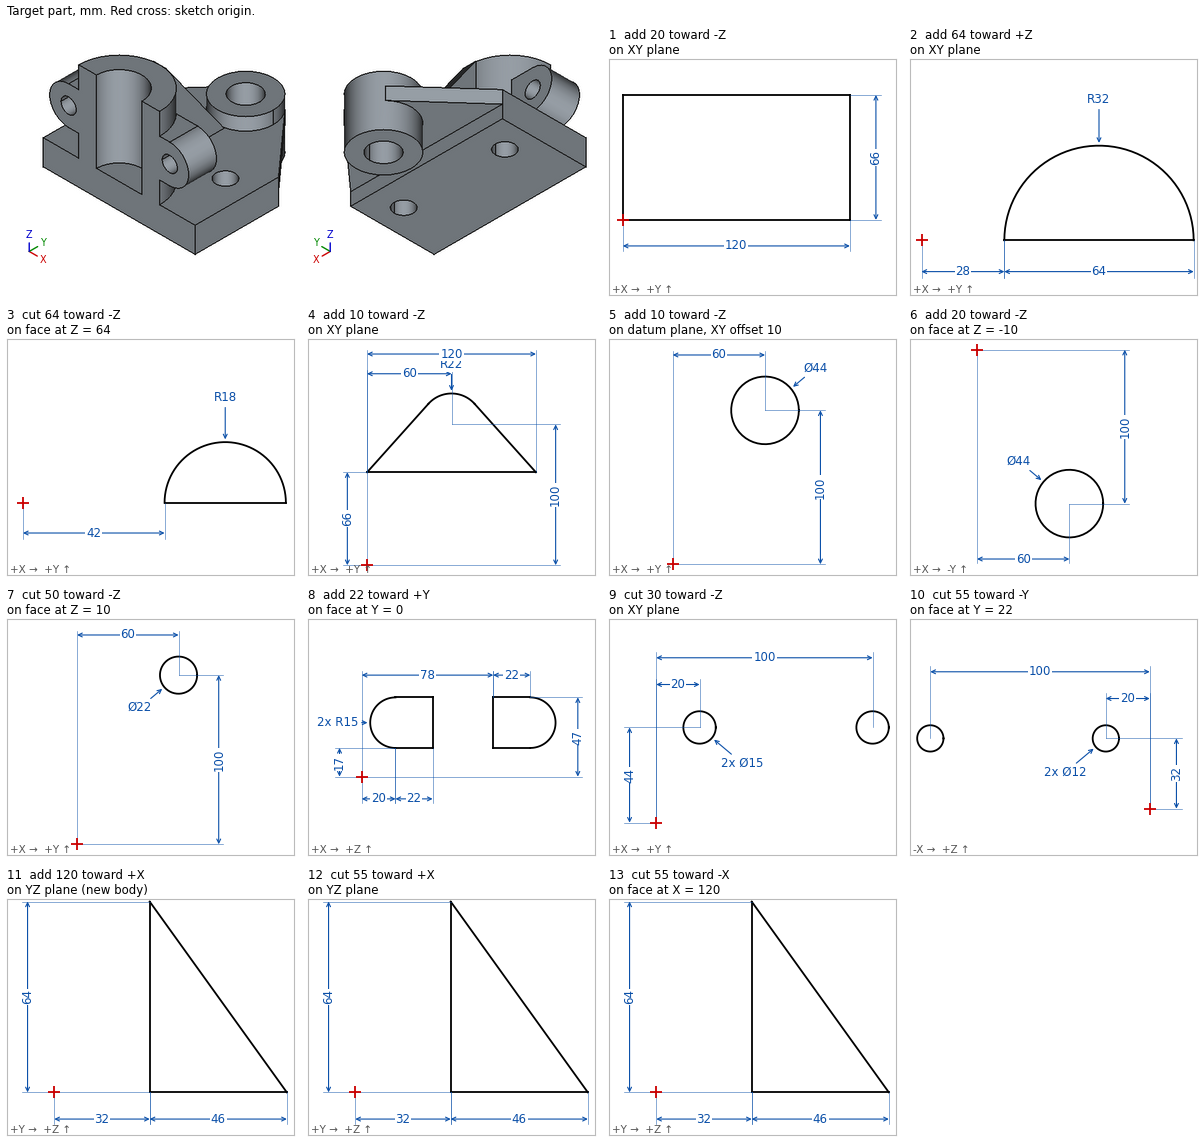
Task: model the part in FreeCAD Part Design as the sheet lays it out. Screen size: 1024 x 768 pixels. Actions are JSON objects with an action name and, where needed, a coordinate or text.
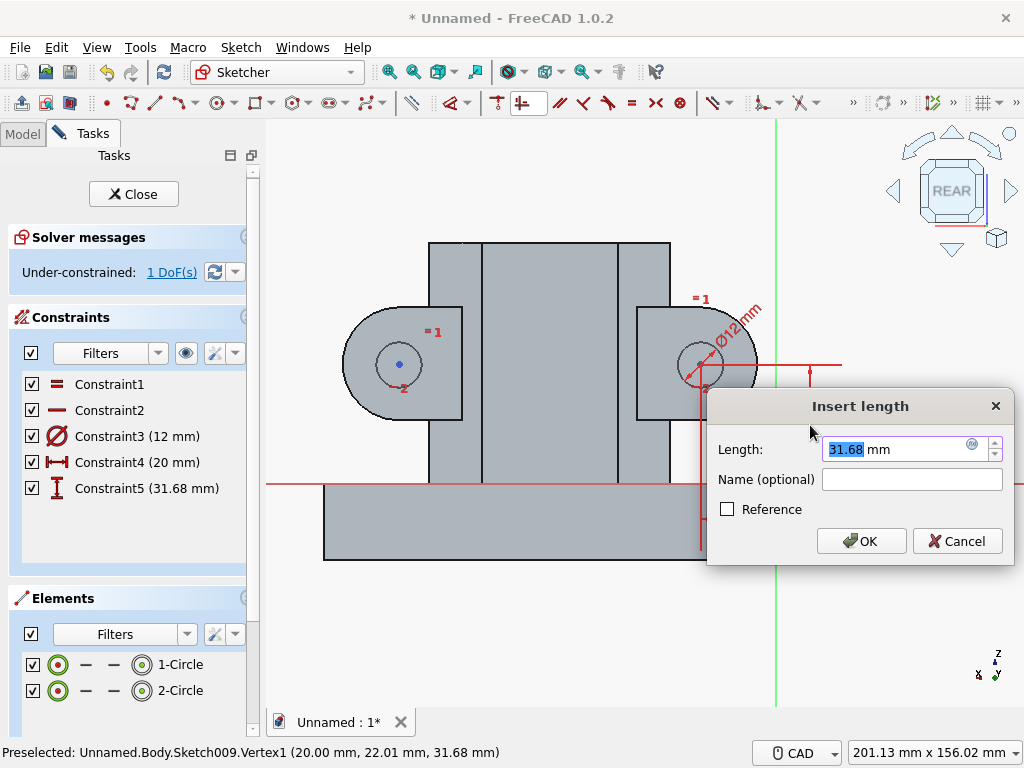
{"action": "type", "text": "32"}
{"action": "key", "text": "Return"}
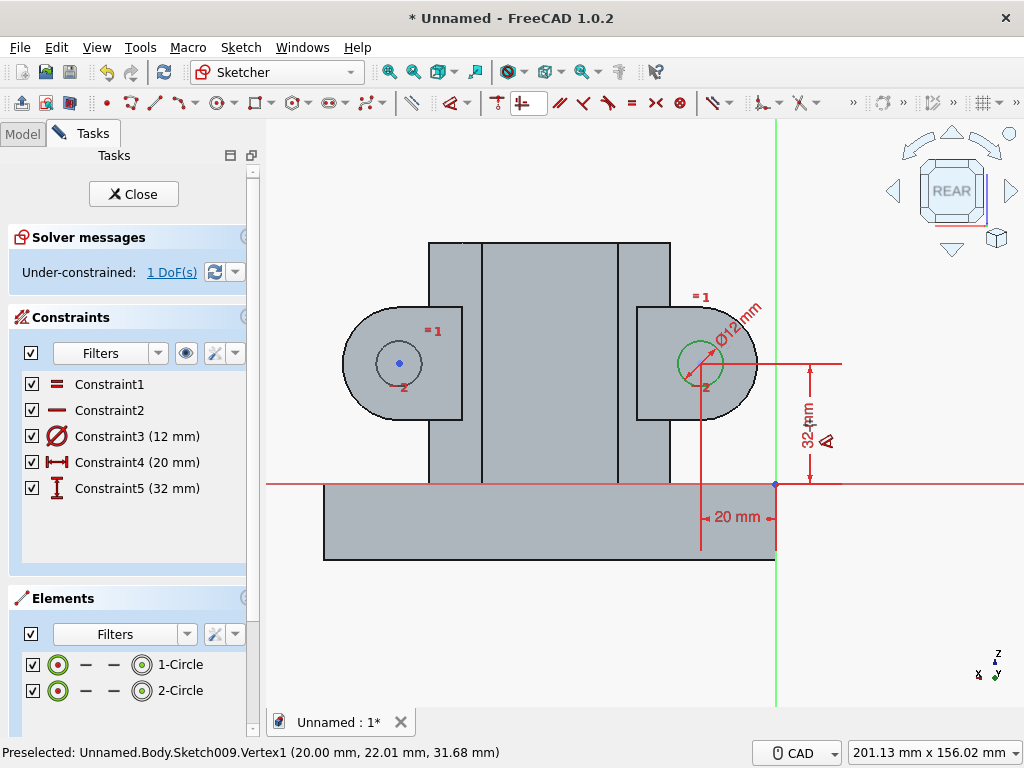
{"action": "left_click", "coordinate": [399, 364]}
{"action": "left_click", "coordinate": [587, 518]}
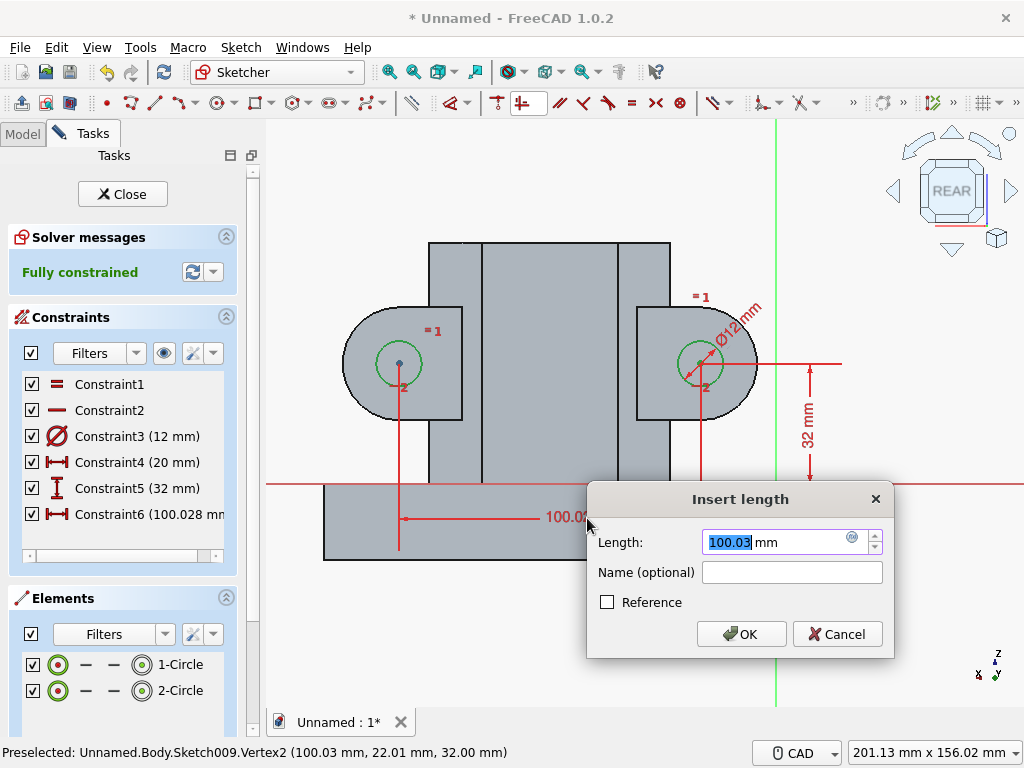
{"action": "type", "text": "100"}
{"action": "key", "text": "Return"}
{"action": "key", "text": "Escape"}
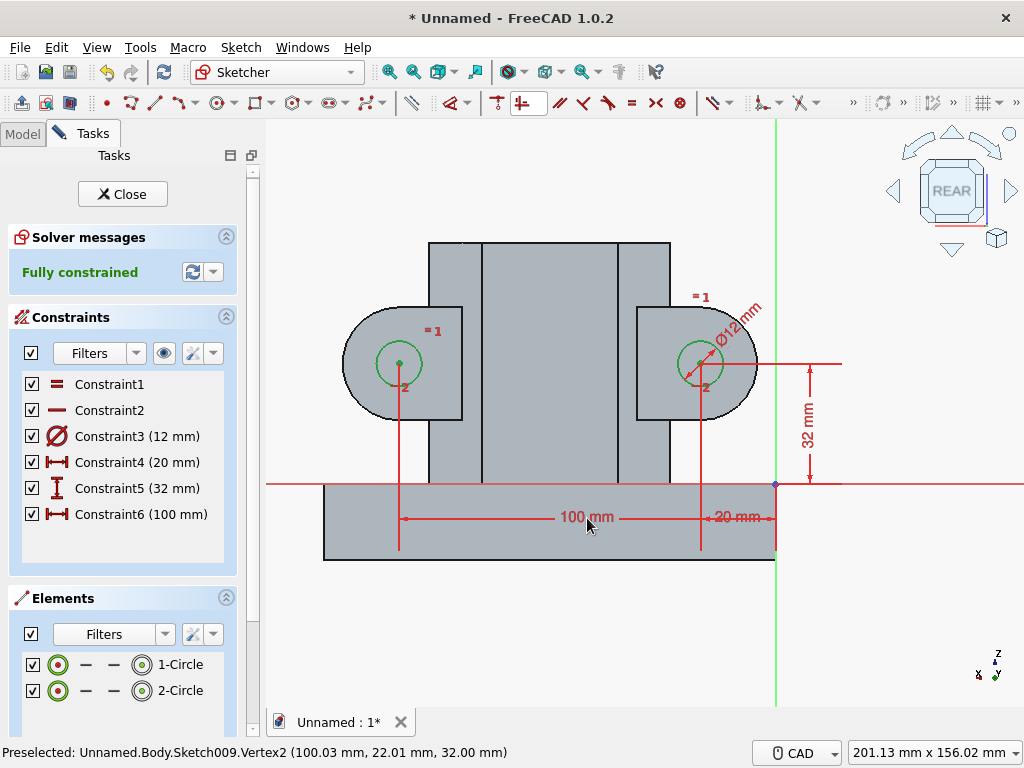
{"action": "left_click", "coordinate": [123, 194]}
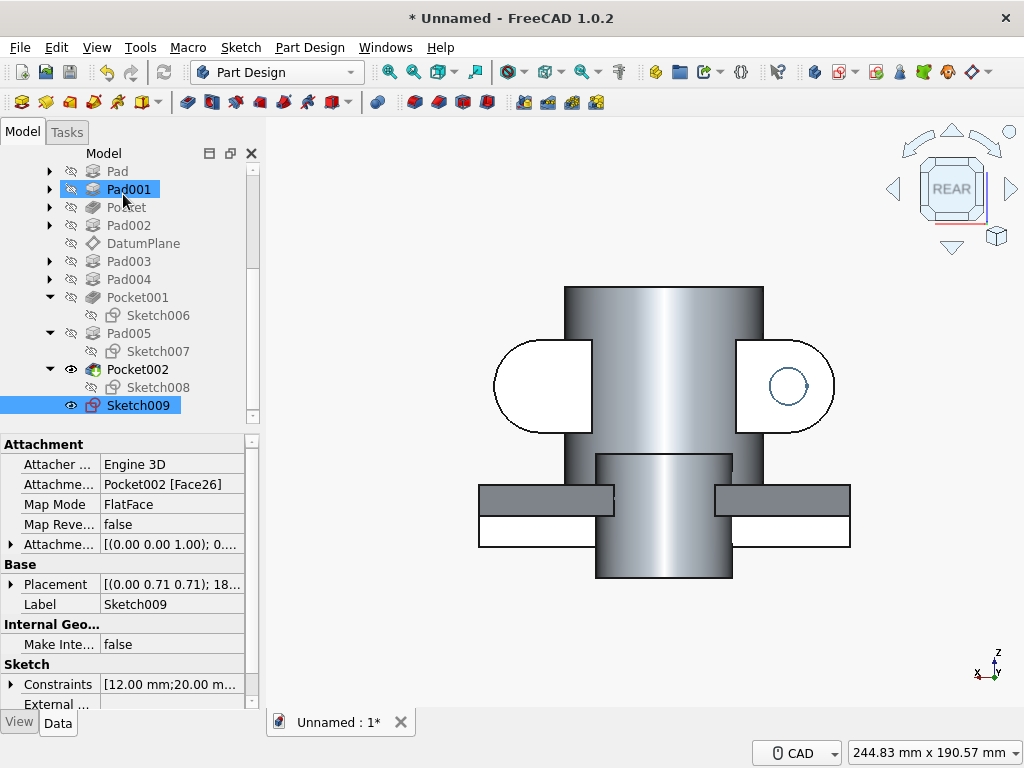
{"action": "left_click", "coordinate": [188, 102]}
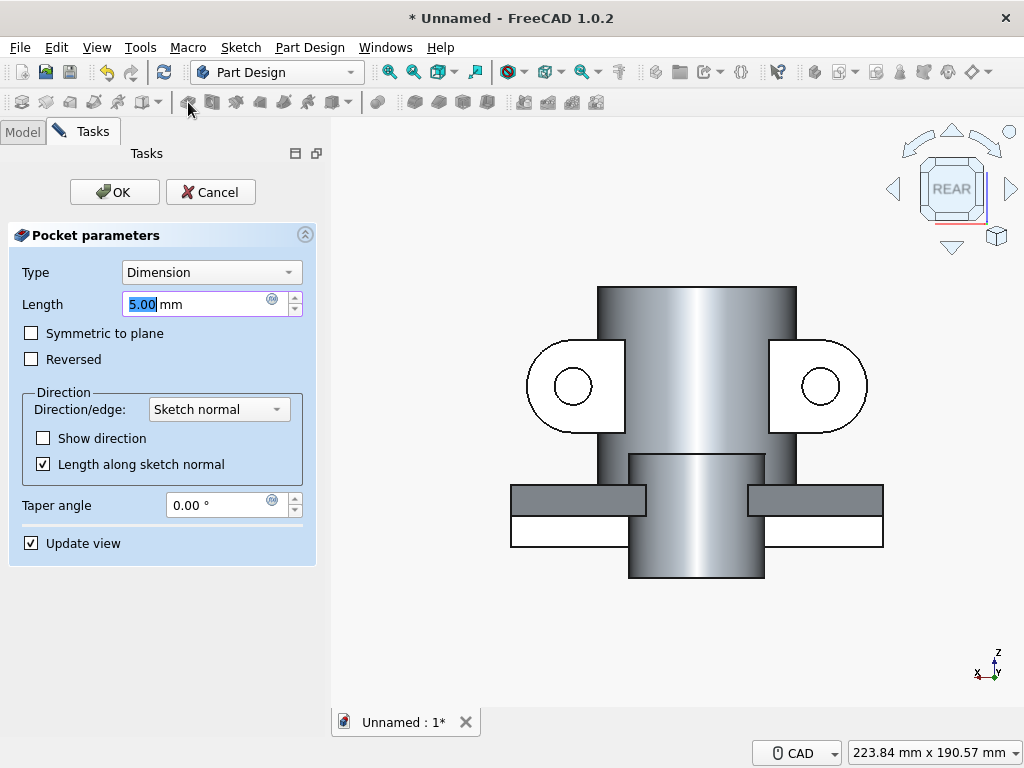
{"action": "type", "text": "55"}
{"action": "key", "text": "Tab"}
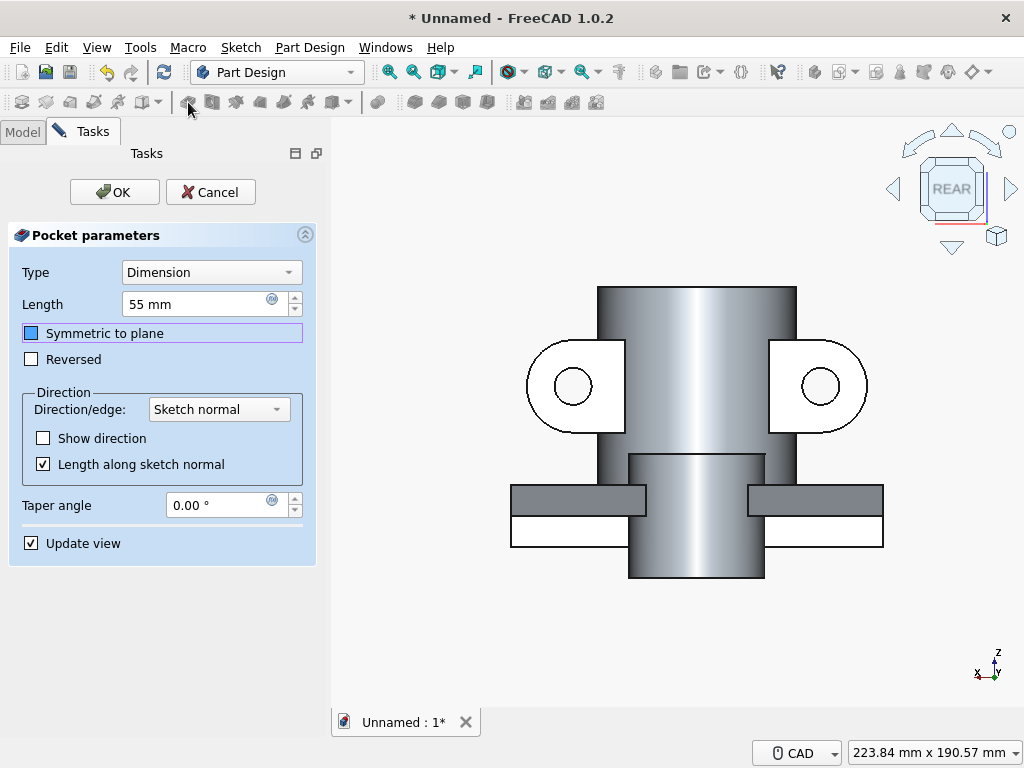
{"action": "left_click", "coordinate": [115, 192]}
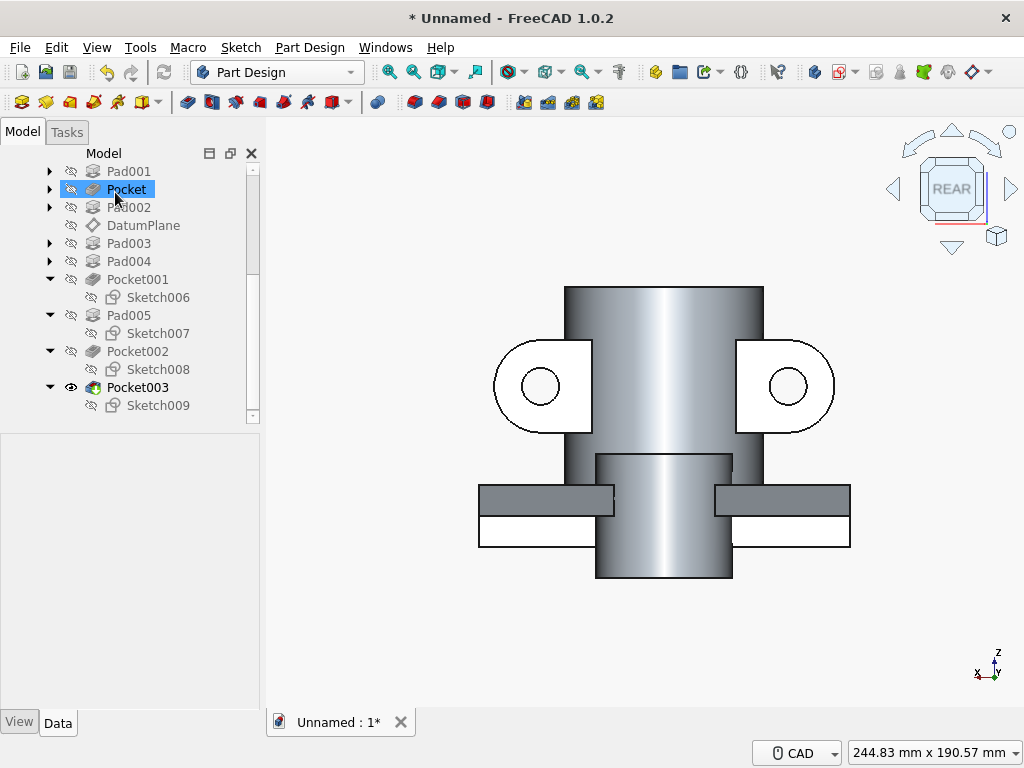
{"action": "left_click", "coordinate": [816, 72]}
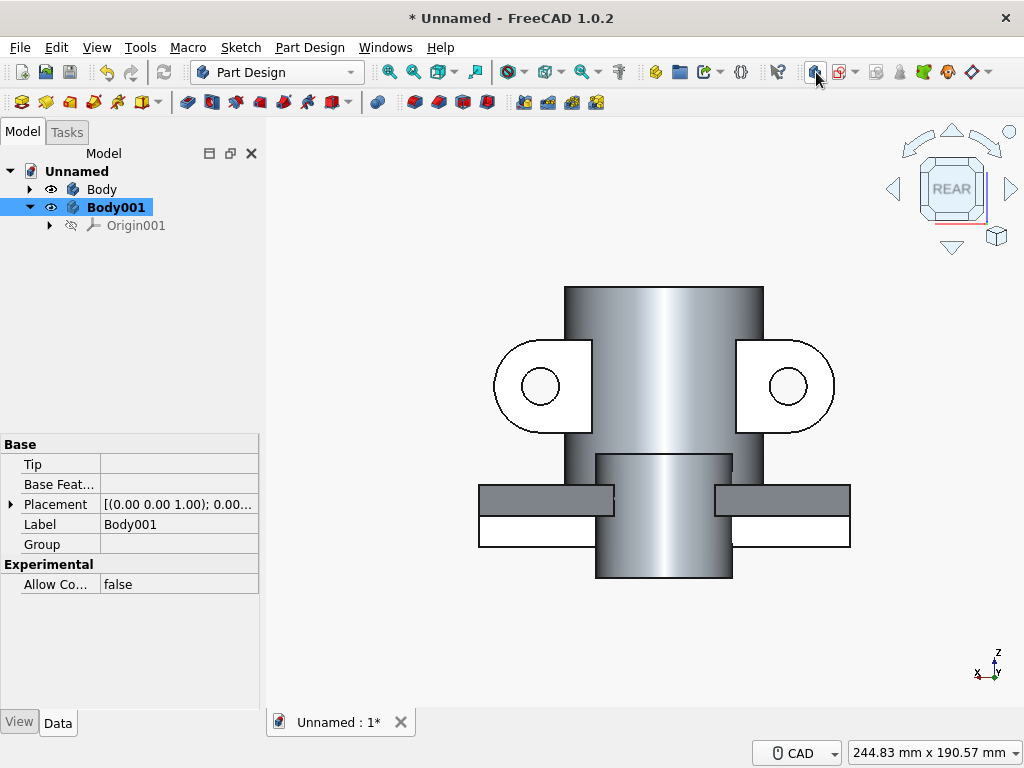
{"action": "left_click", "coordinate": [306, 667]}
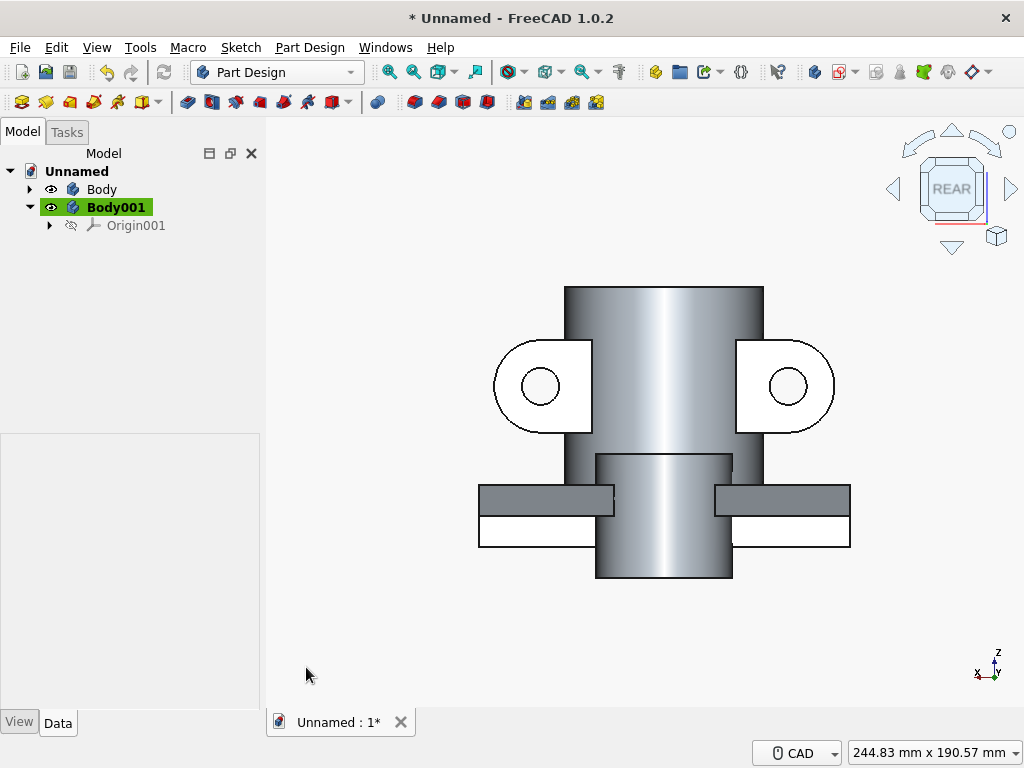
{"action": "left_click", "coordinate": [840, 72]}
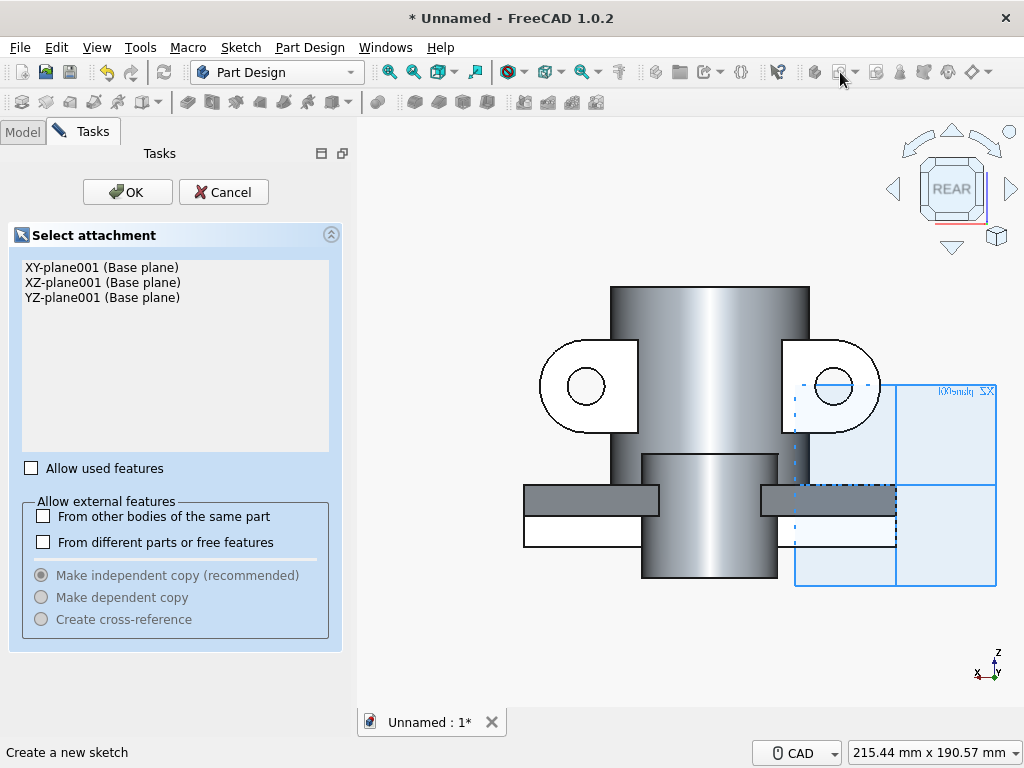
{"action": "left_click", "coordinate": [82, 298]}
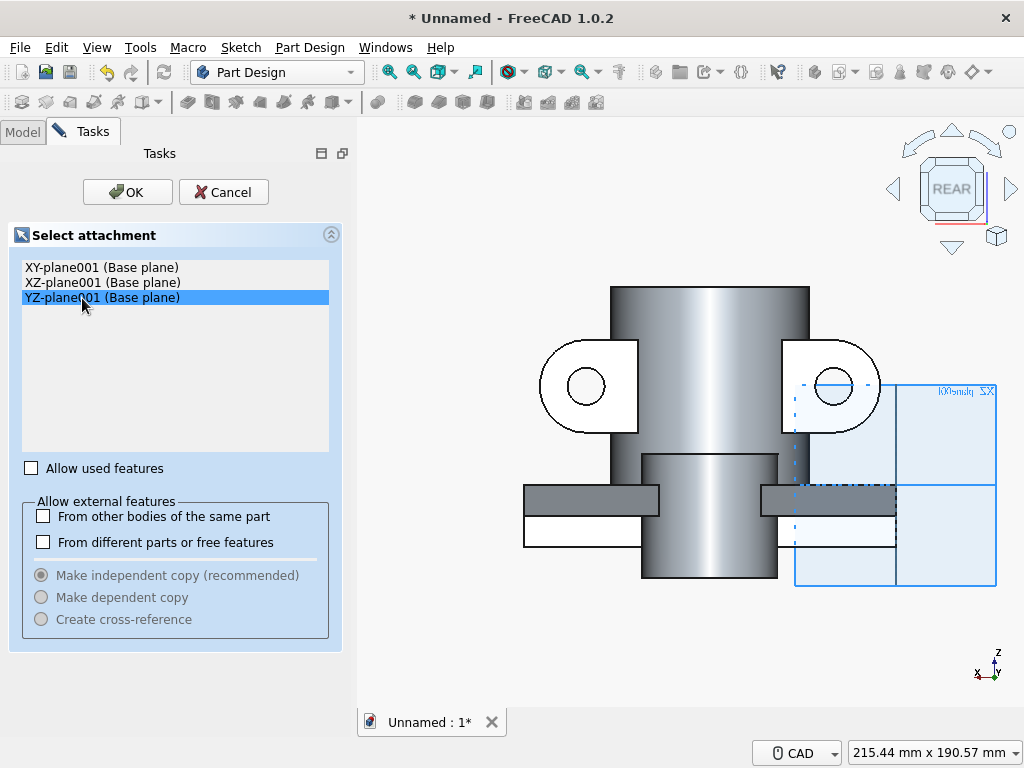
{"action": "left_click", "coordinate": [128, 192]}